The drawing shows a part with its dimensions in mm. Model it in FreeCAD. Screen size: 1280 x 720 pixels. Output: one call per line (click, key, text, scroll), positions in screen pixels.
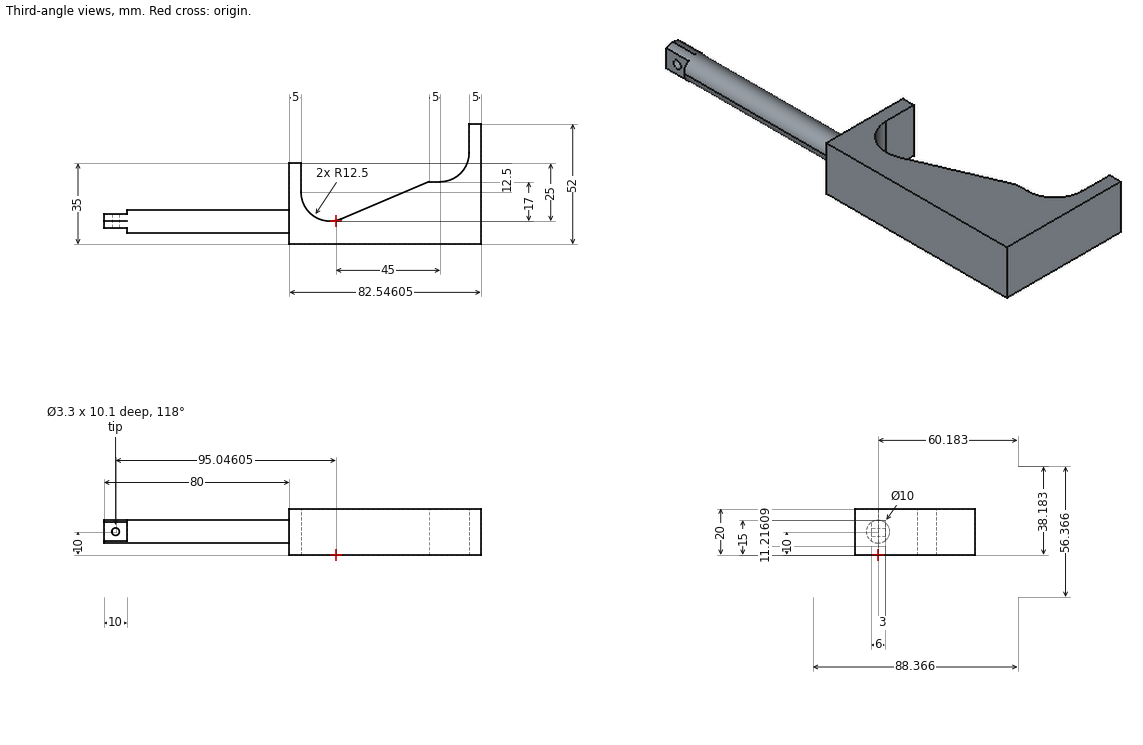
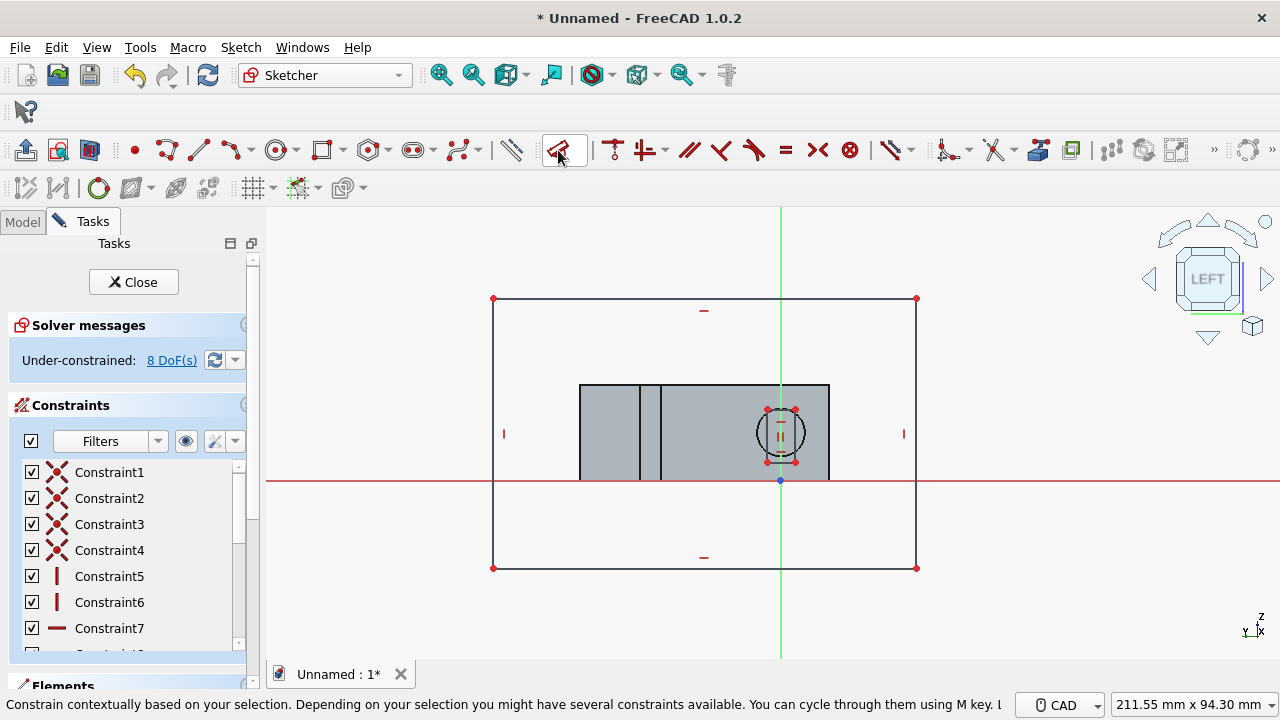
scroll(778, 463, up, 2)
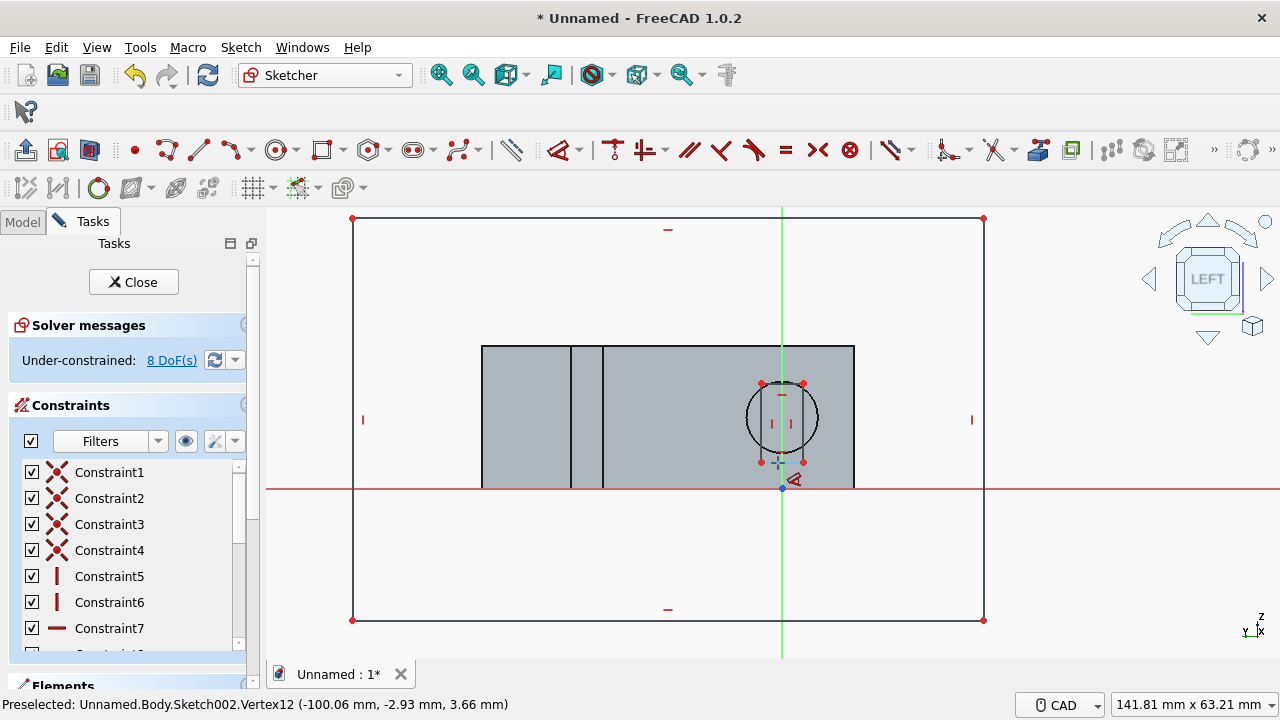
click(778, 463)
click(768, 521)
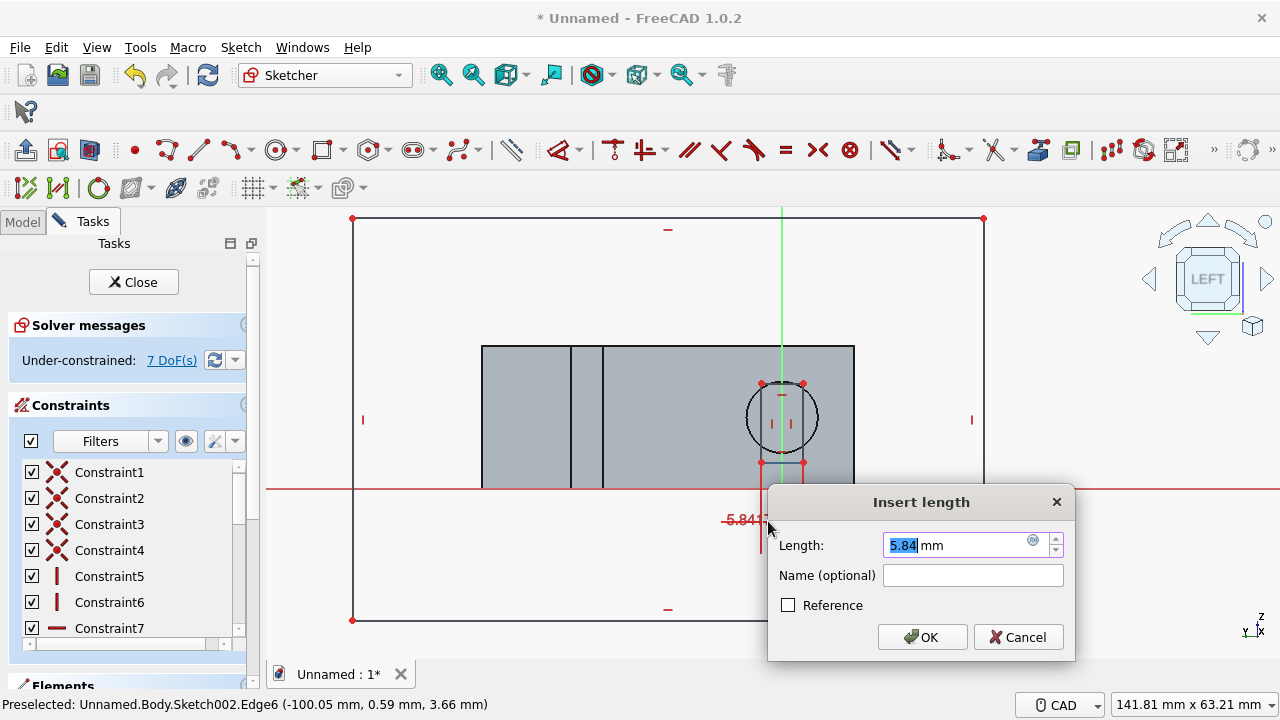
text(6)
key(Return)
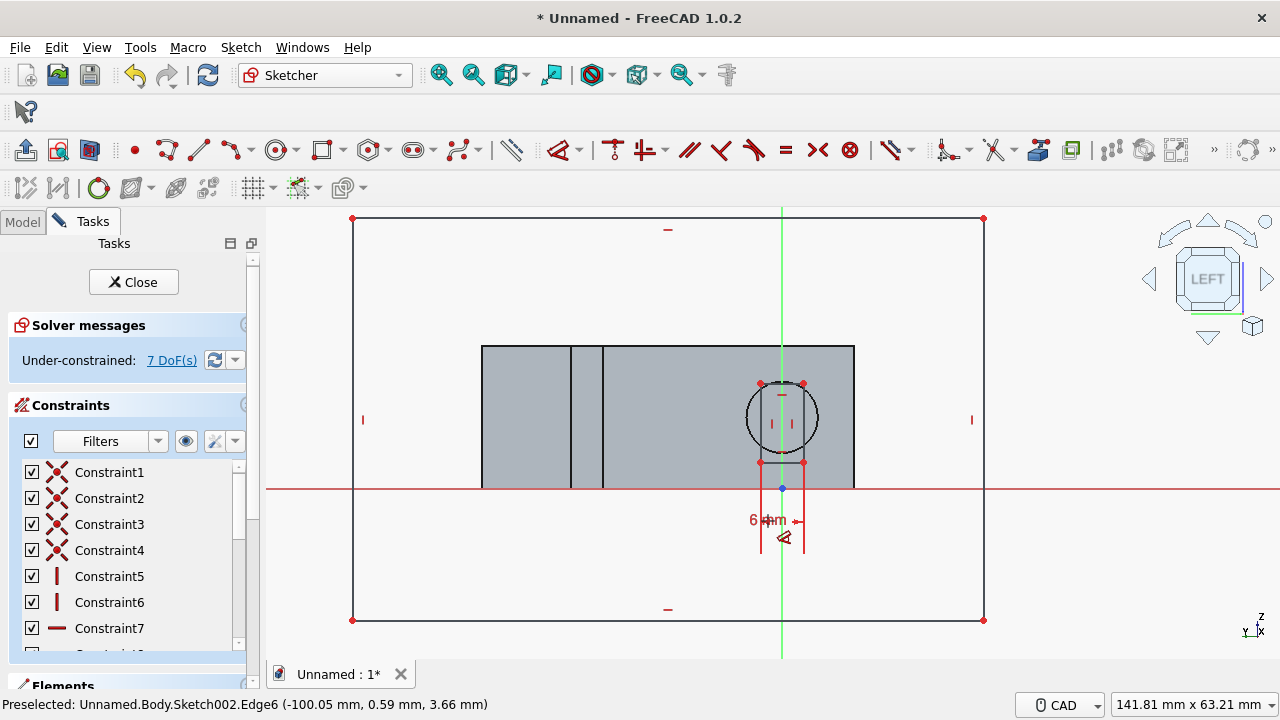
scroll(761, 384, up, 4)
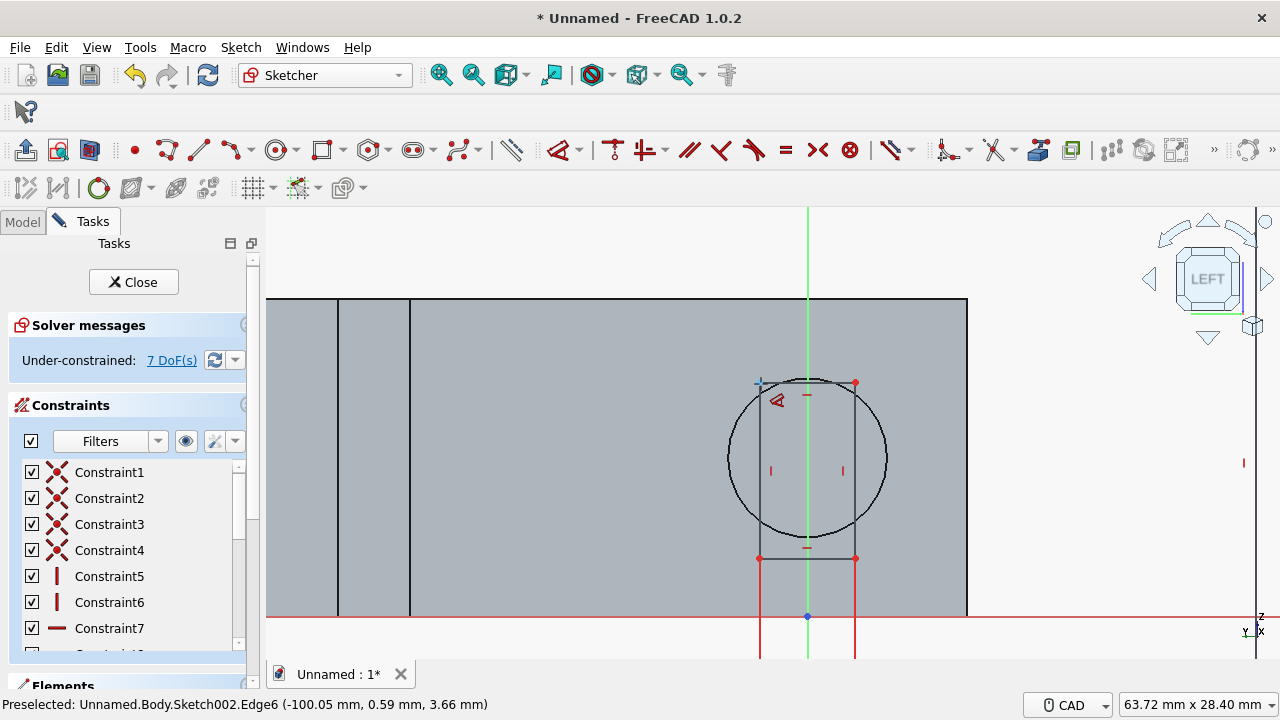
click(760, 383)
click(784, 349)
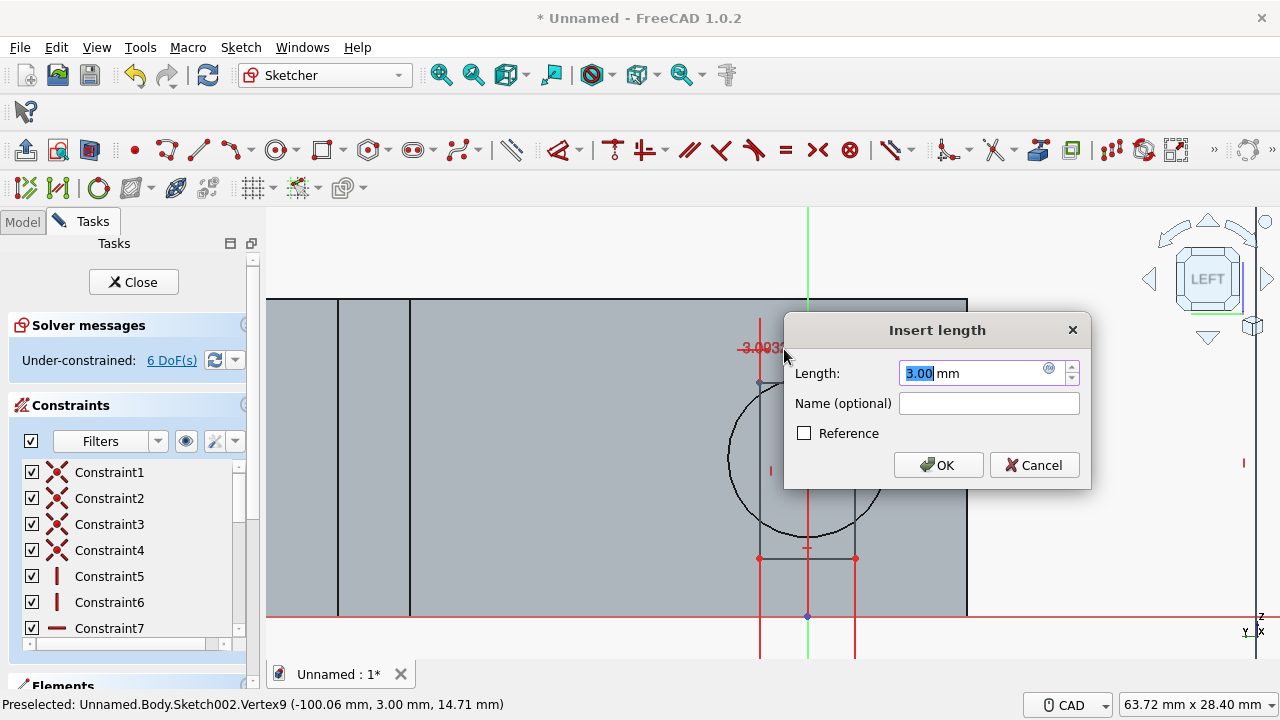
text(3)
key(Return)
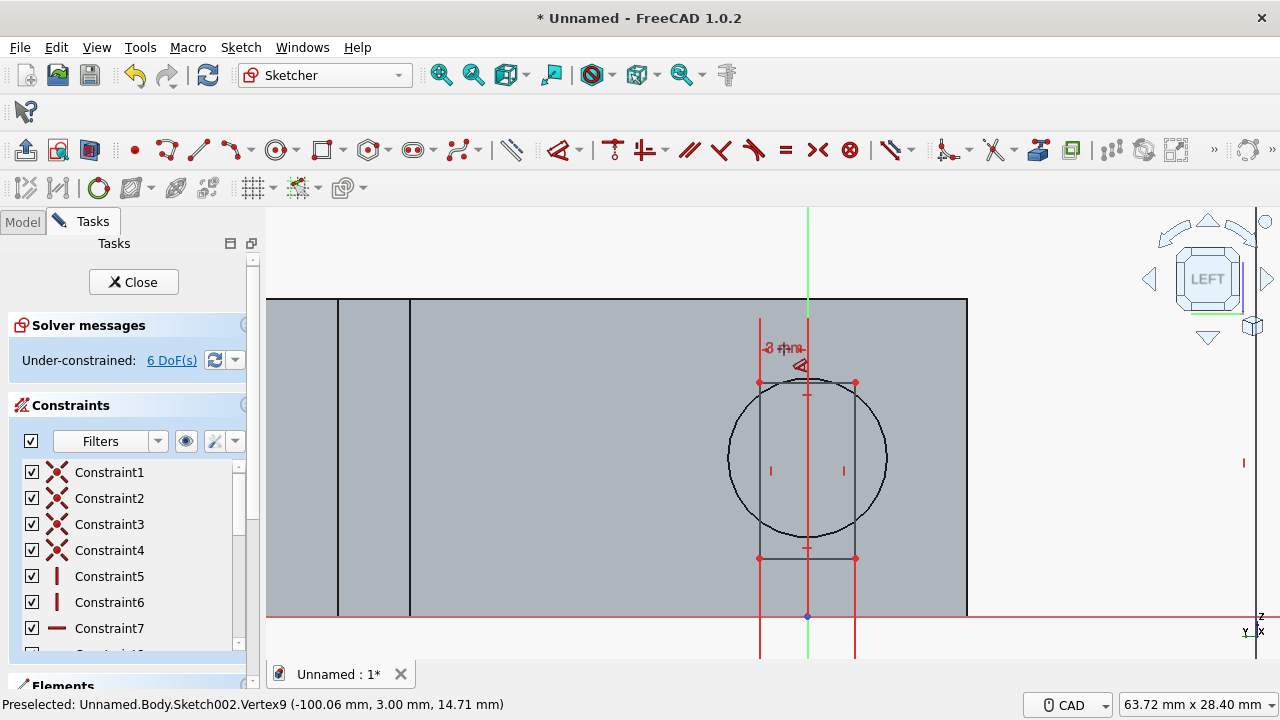
click(760, 383)
click(842, 500)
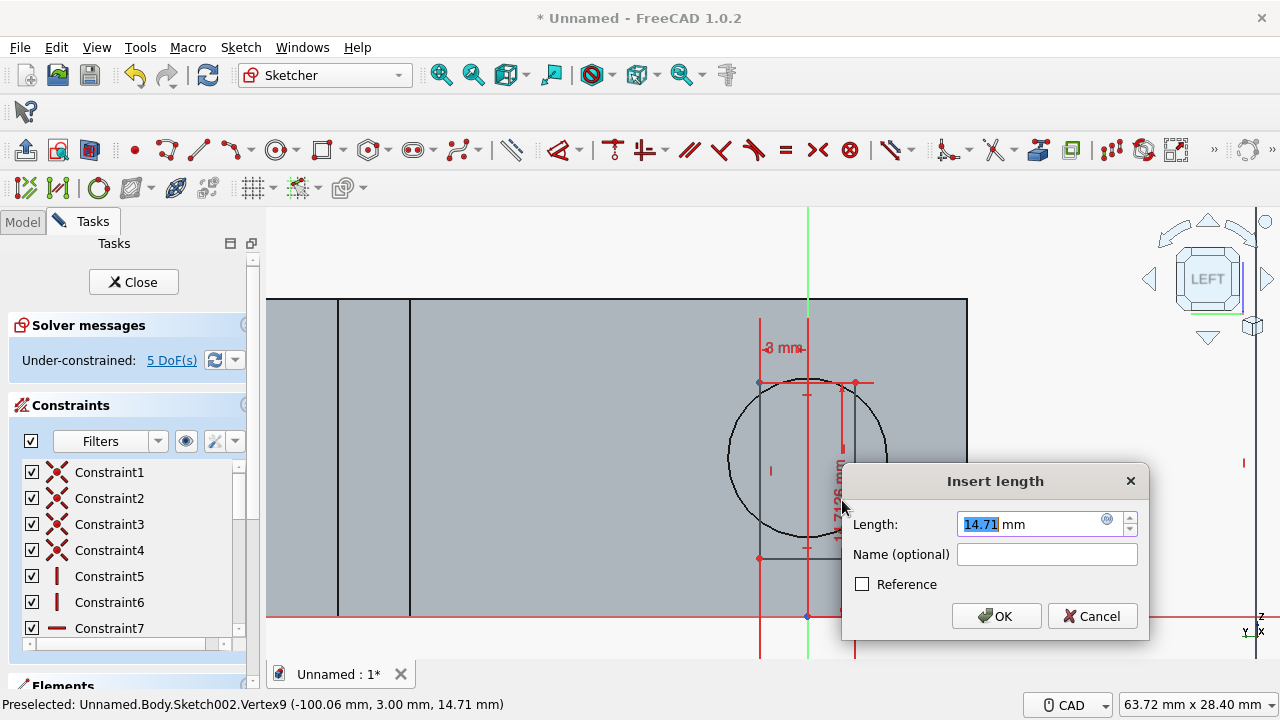
text(15)
key(Return)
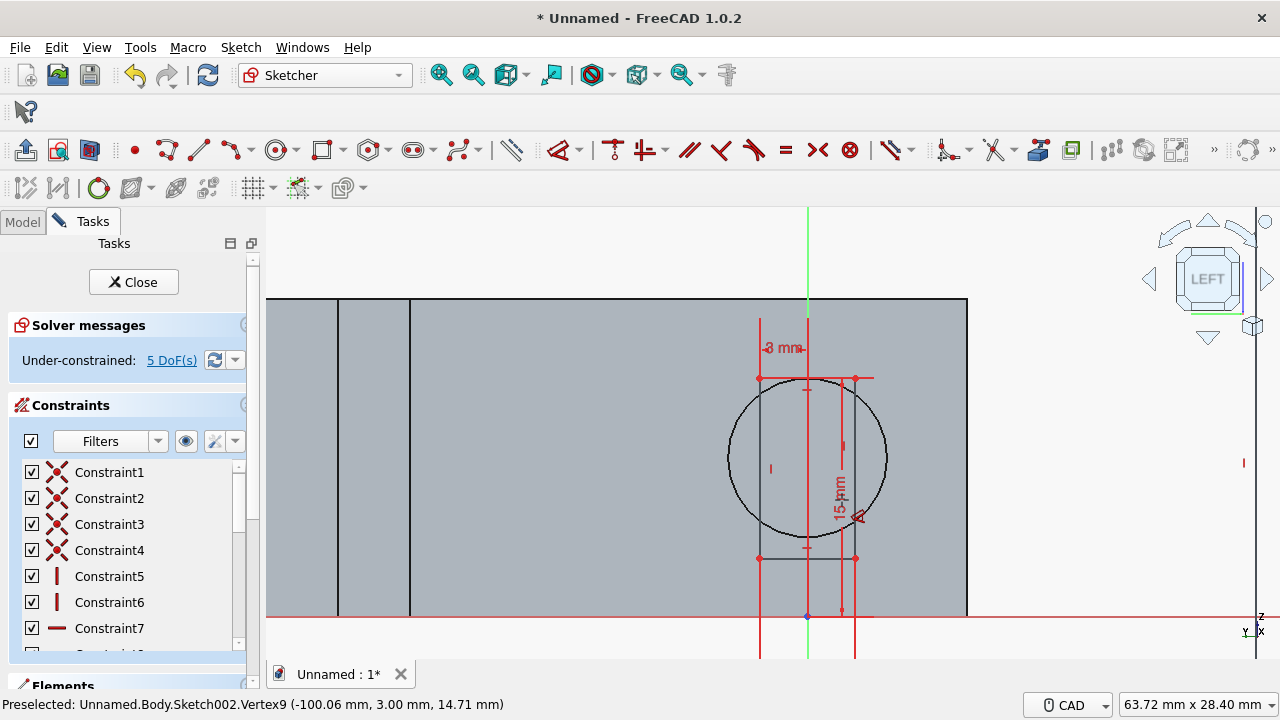
scroll(770, 422, down, 6)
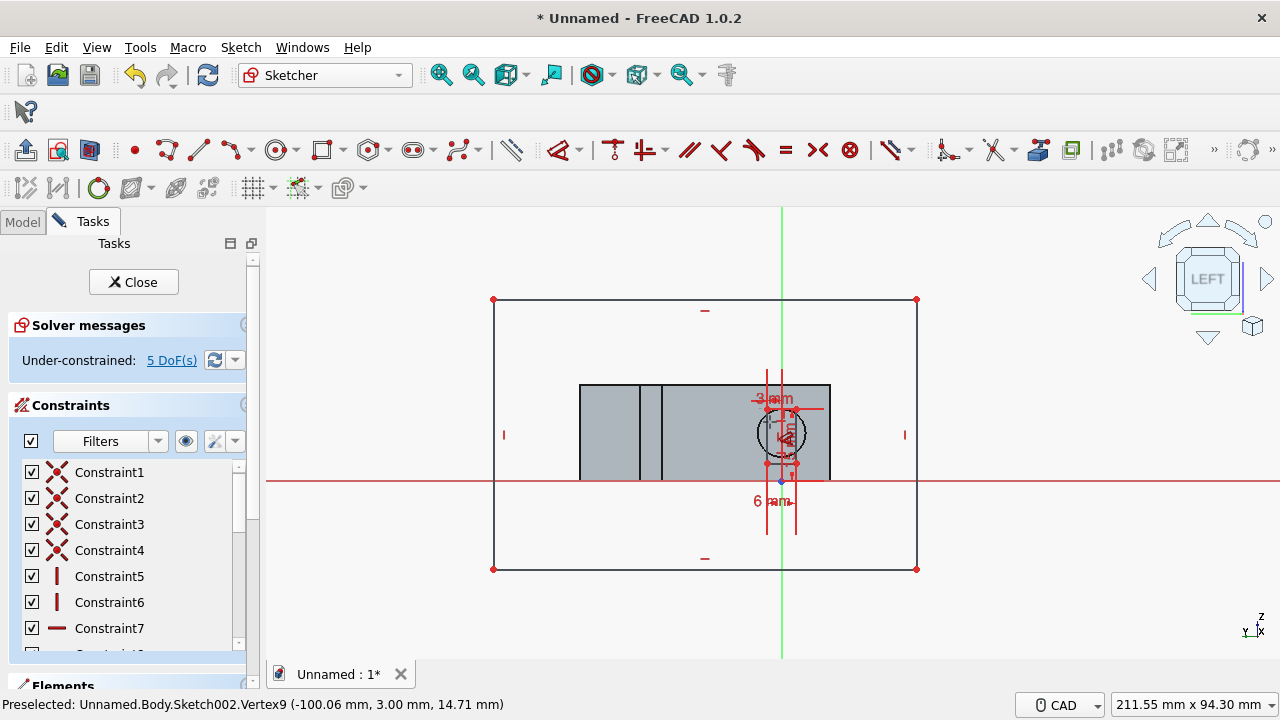
click(494, 381)
click(460, 435)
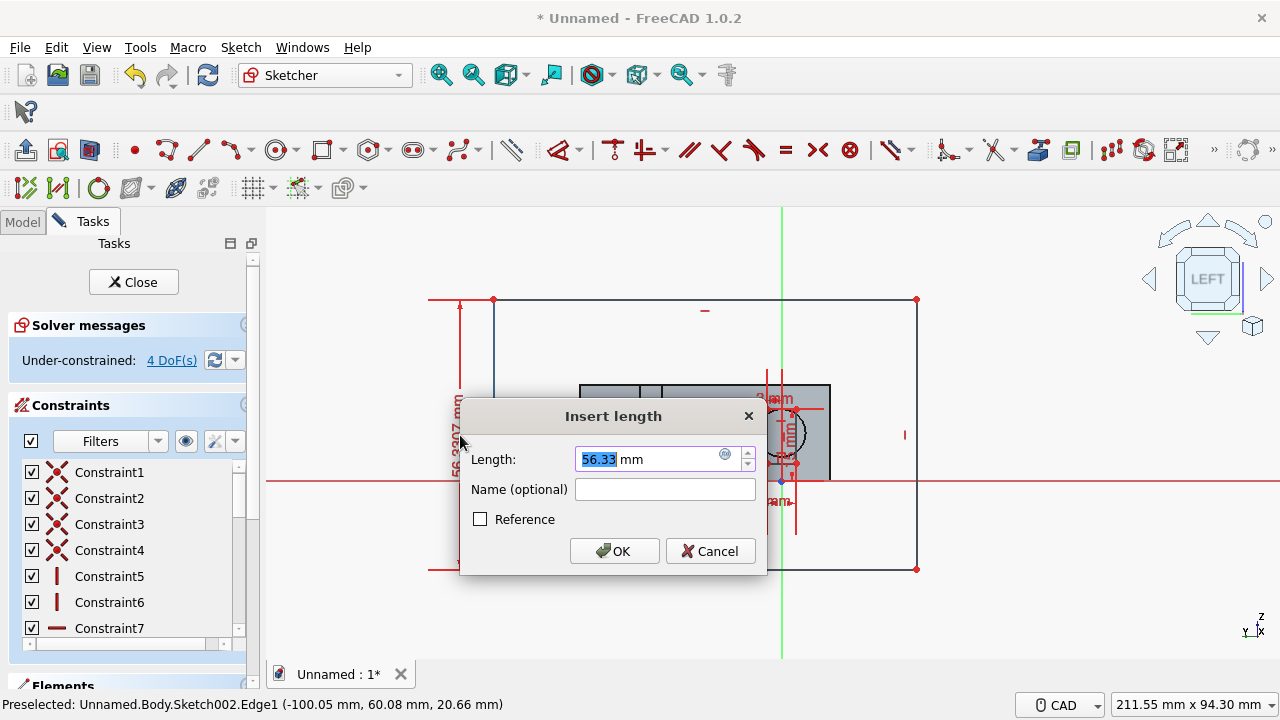
text(56.366)
key(Return)